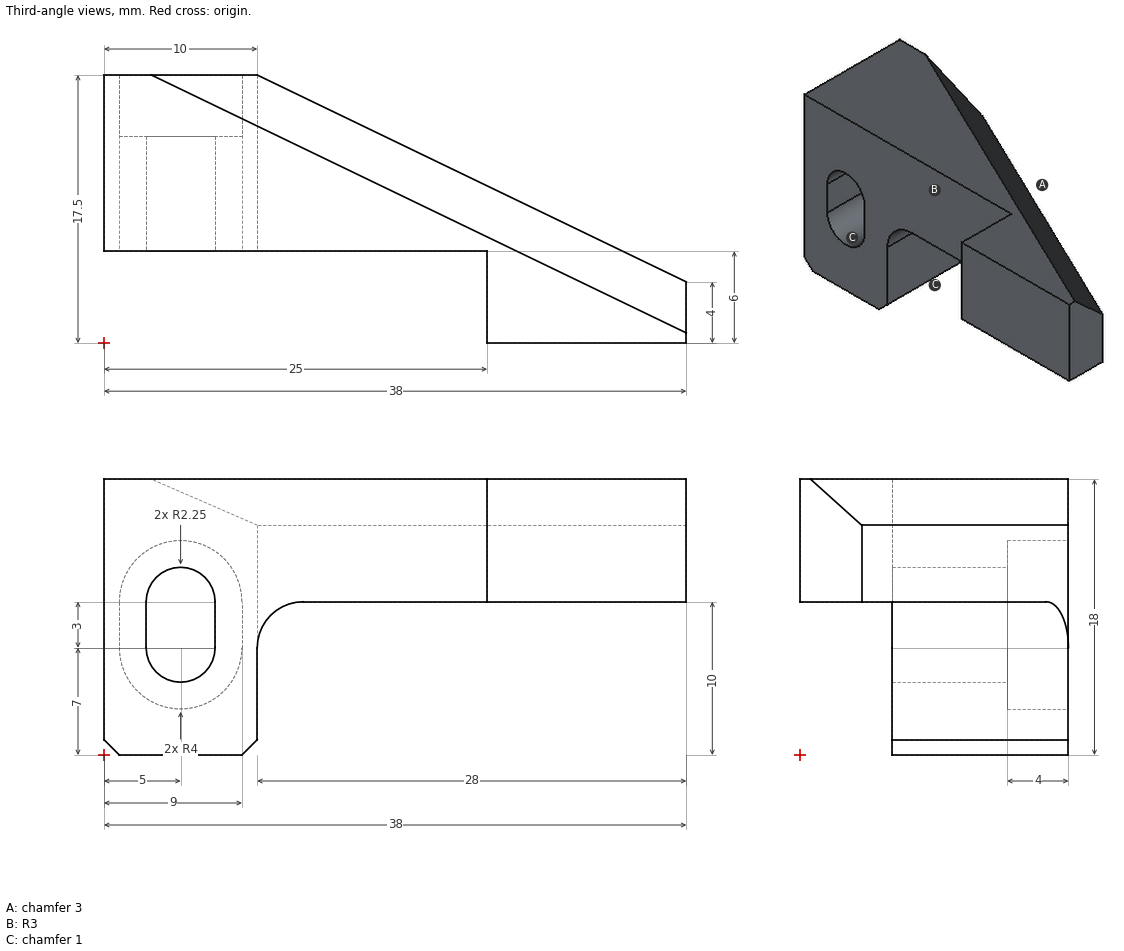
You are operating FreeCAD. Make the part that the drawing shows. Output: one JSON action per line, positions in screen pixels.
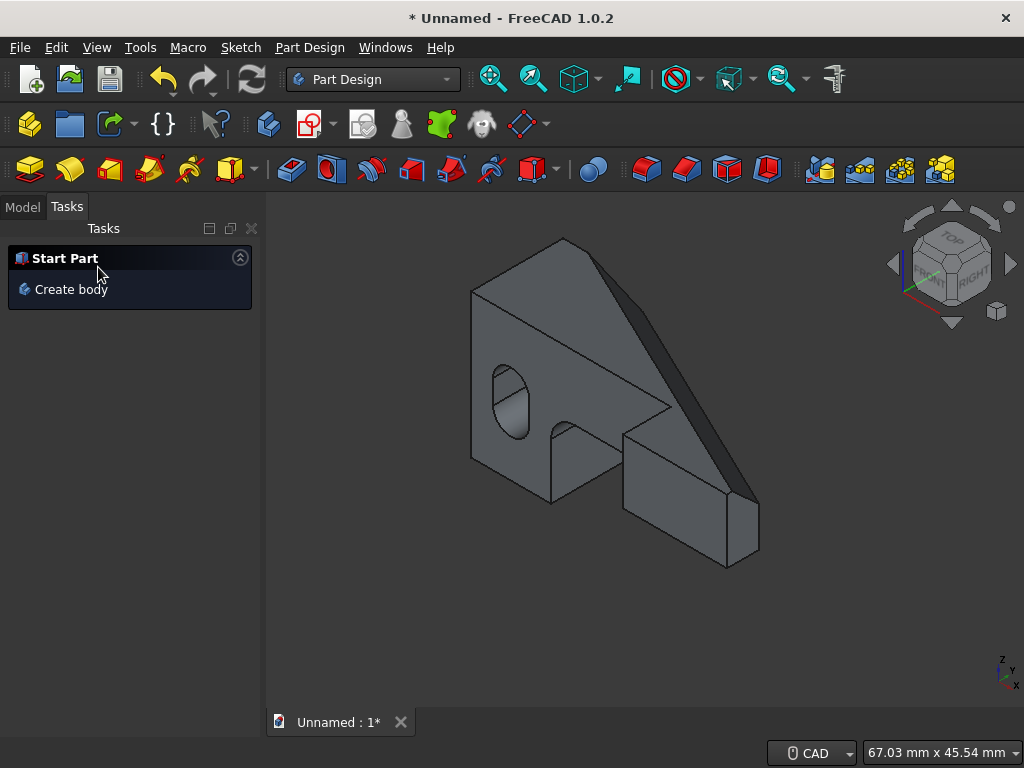
{"action": "key", "text": "1"}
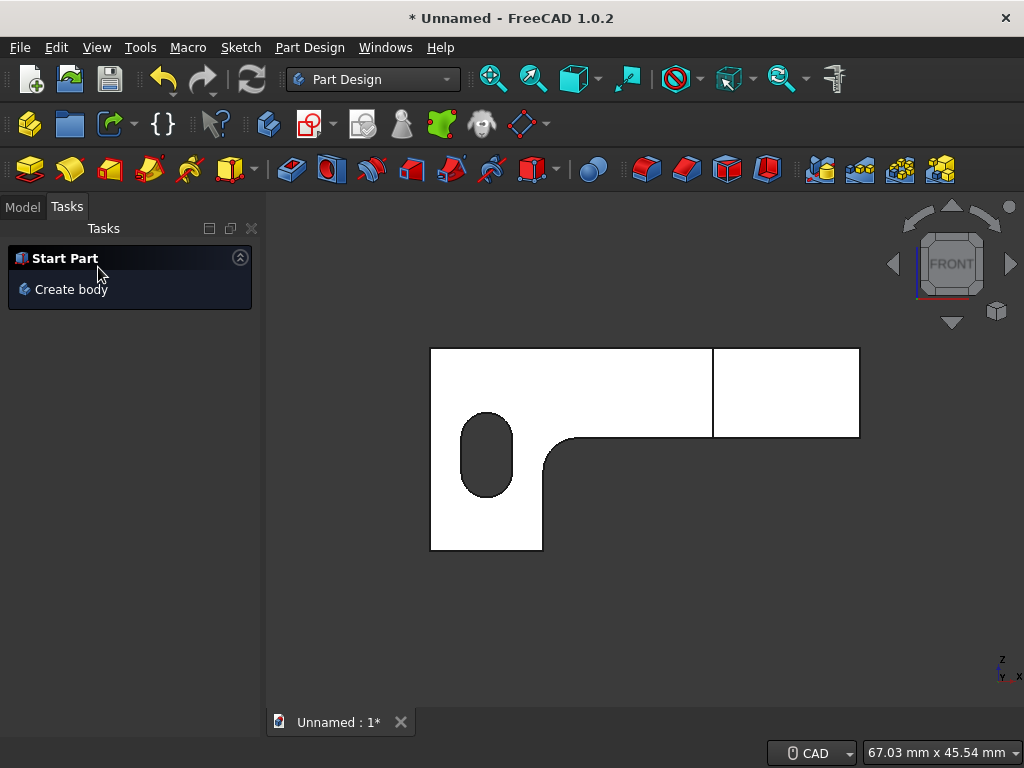
{"action": "key", "text": "3"}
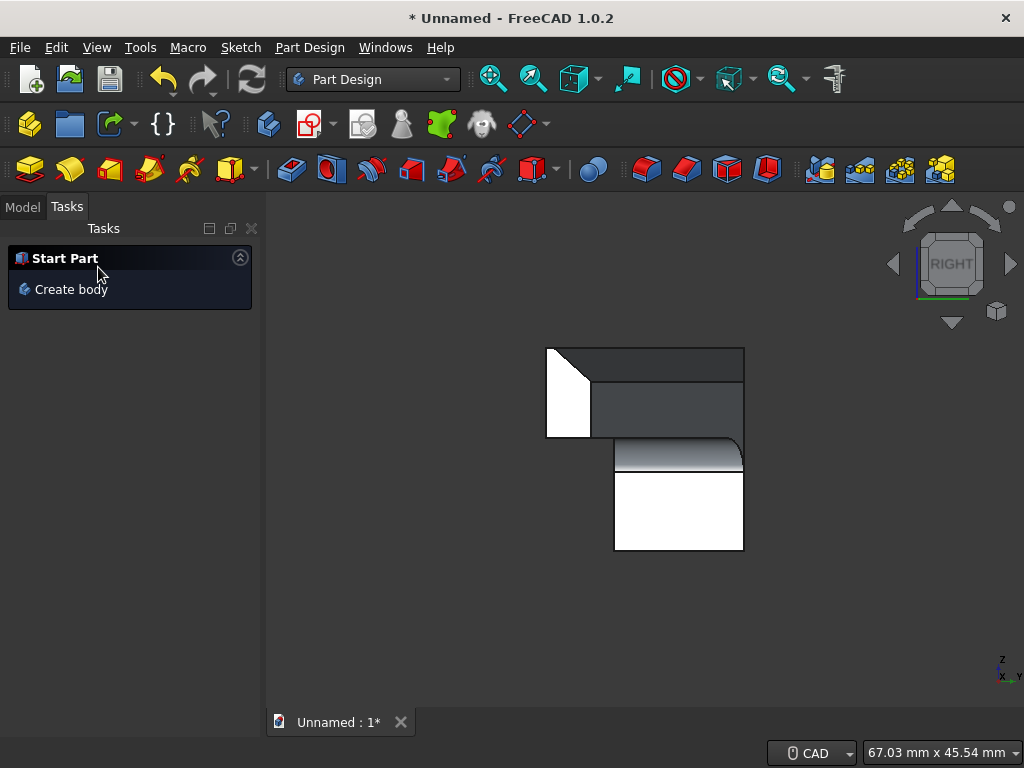
{"action": "key", "text": "v f"}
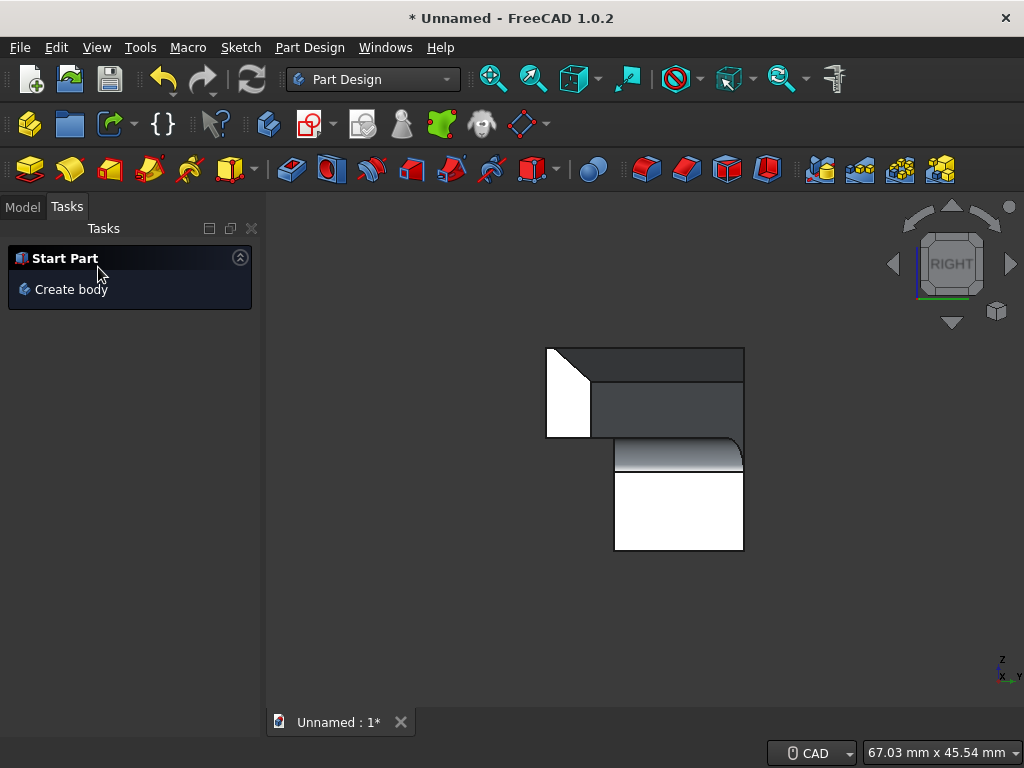
{"action": "left_click", "coordinate": [679, 550]}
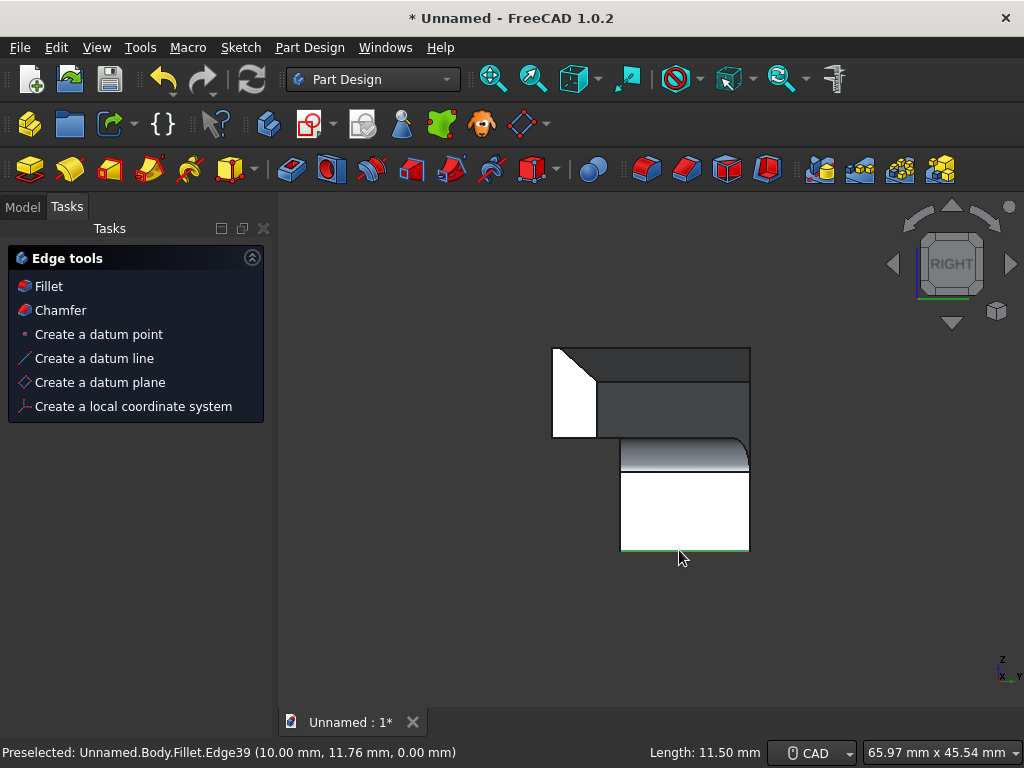
{"action": "key", "text": "5"}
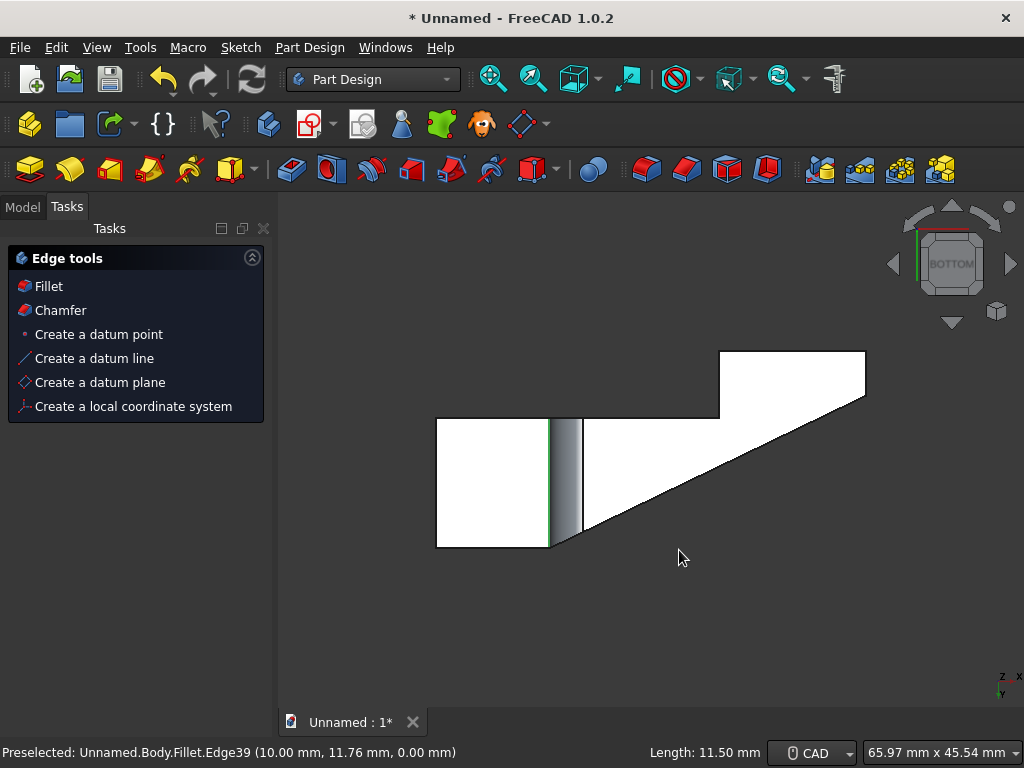
{"action": "left_click", "coordinate": [436, 482], "text": "ctrl"}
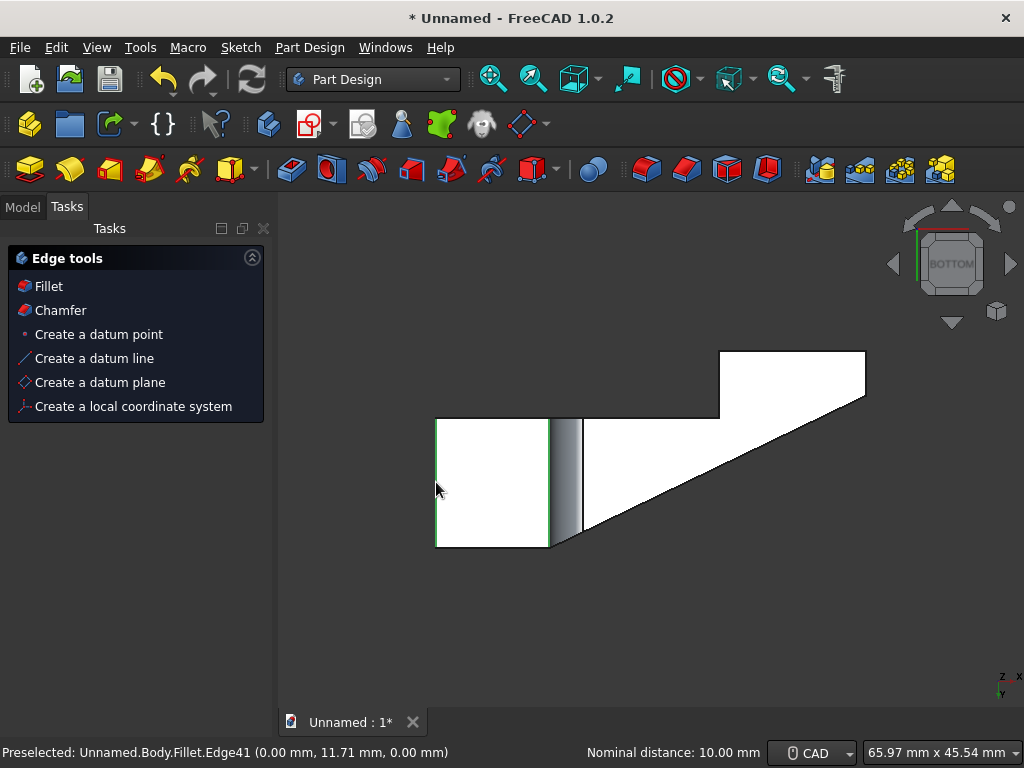
{"action": "left_click", "coordinate": [688, 170]}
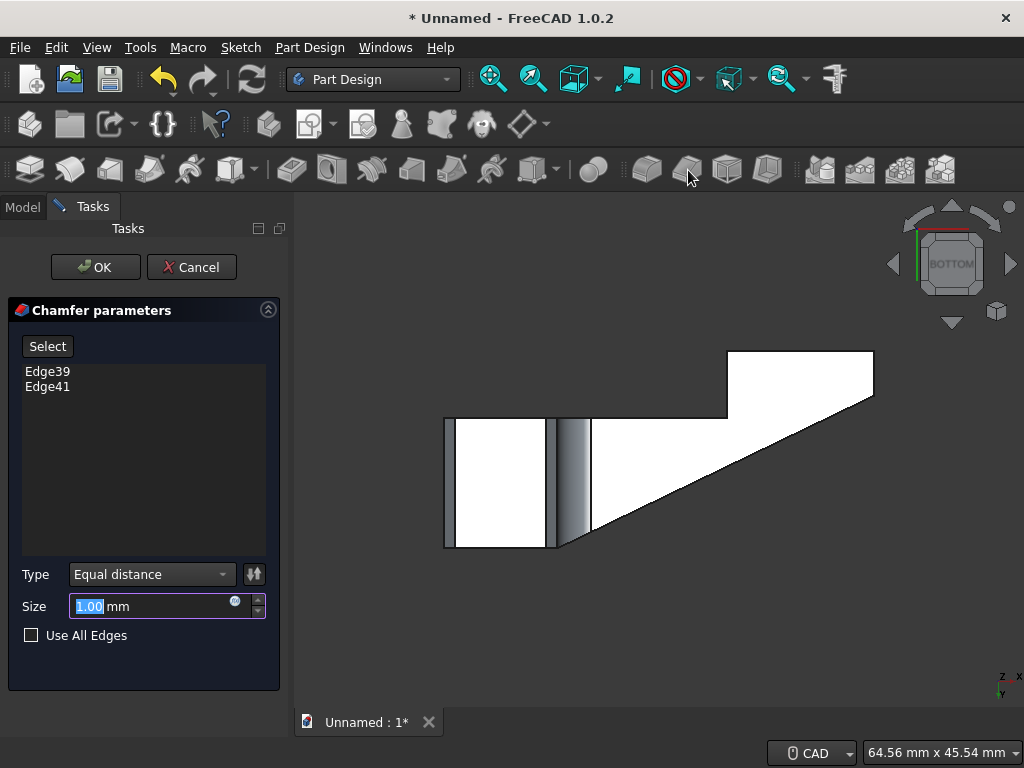
{"action": "type", "text": "1"}
{"action": "key", "text": "Tab"}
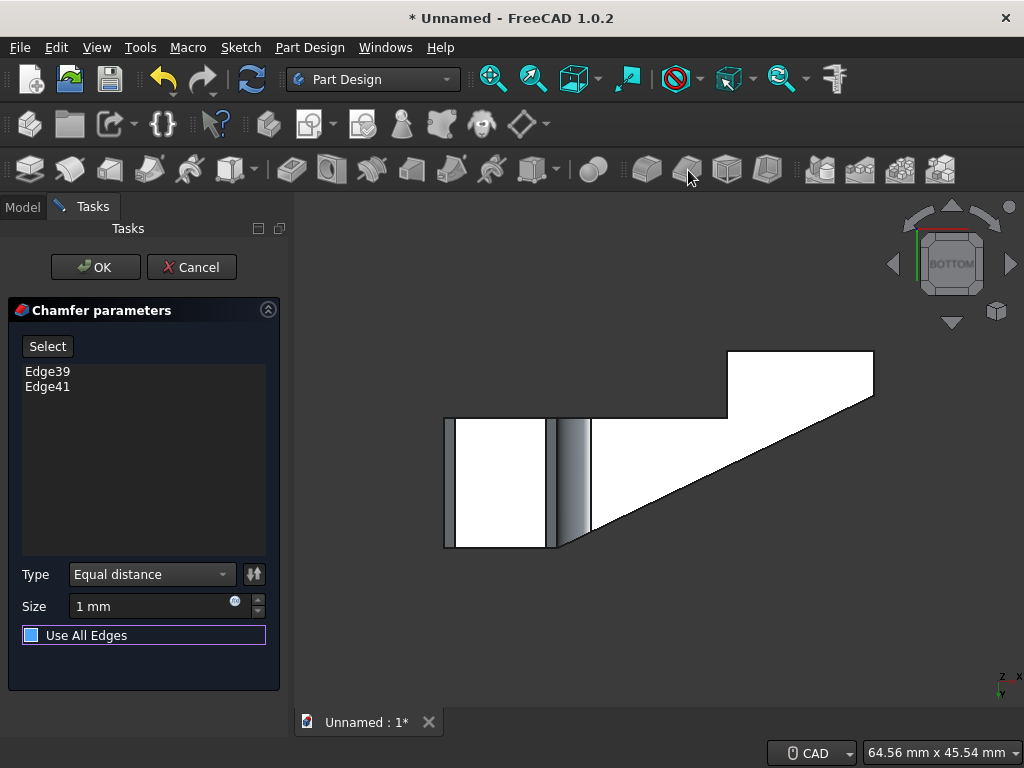
{"action": "left_click", "coordinate": [96, 267]}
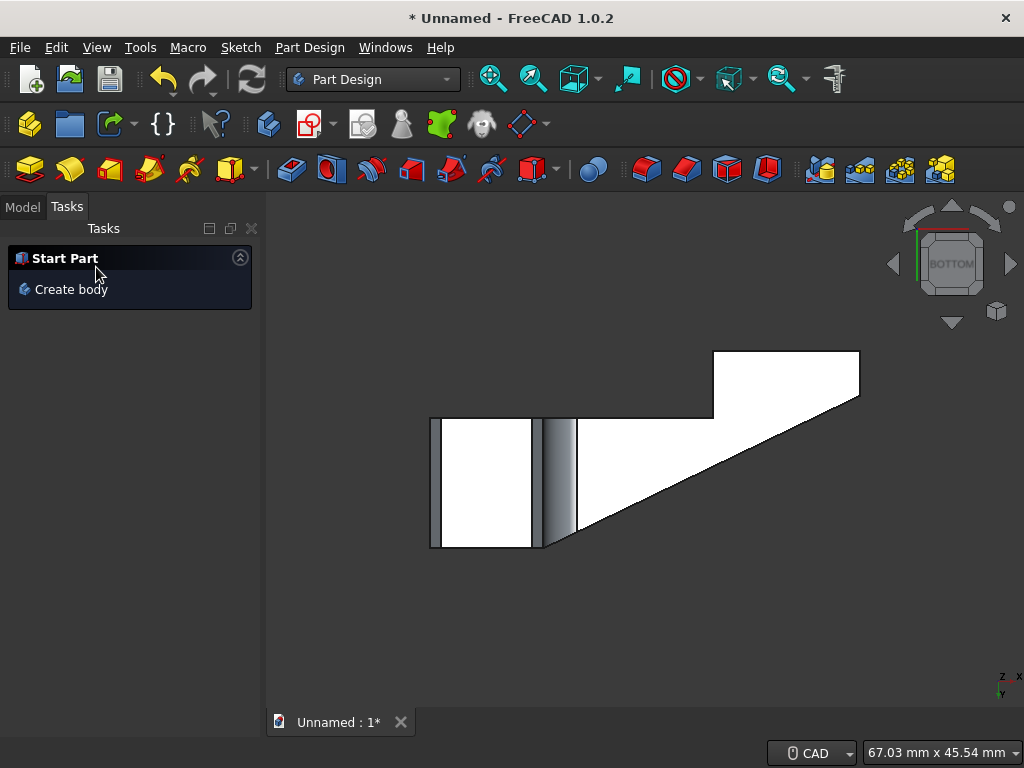
{"action": "key", "text": "0"}